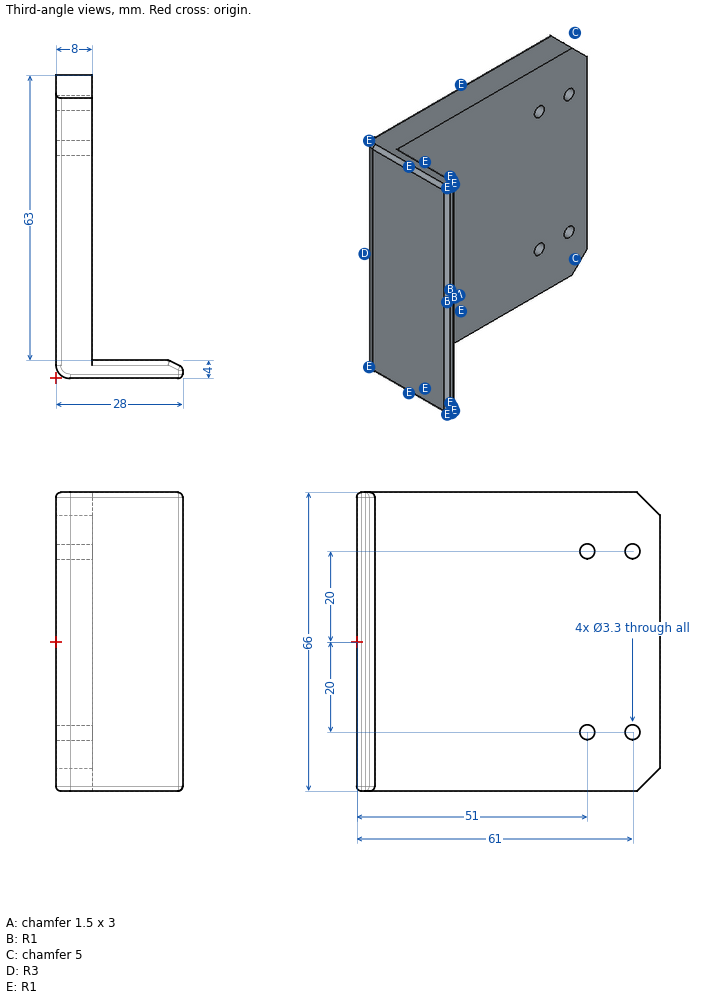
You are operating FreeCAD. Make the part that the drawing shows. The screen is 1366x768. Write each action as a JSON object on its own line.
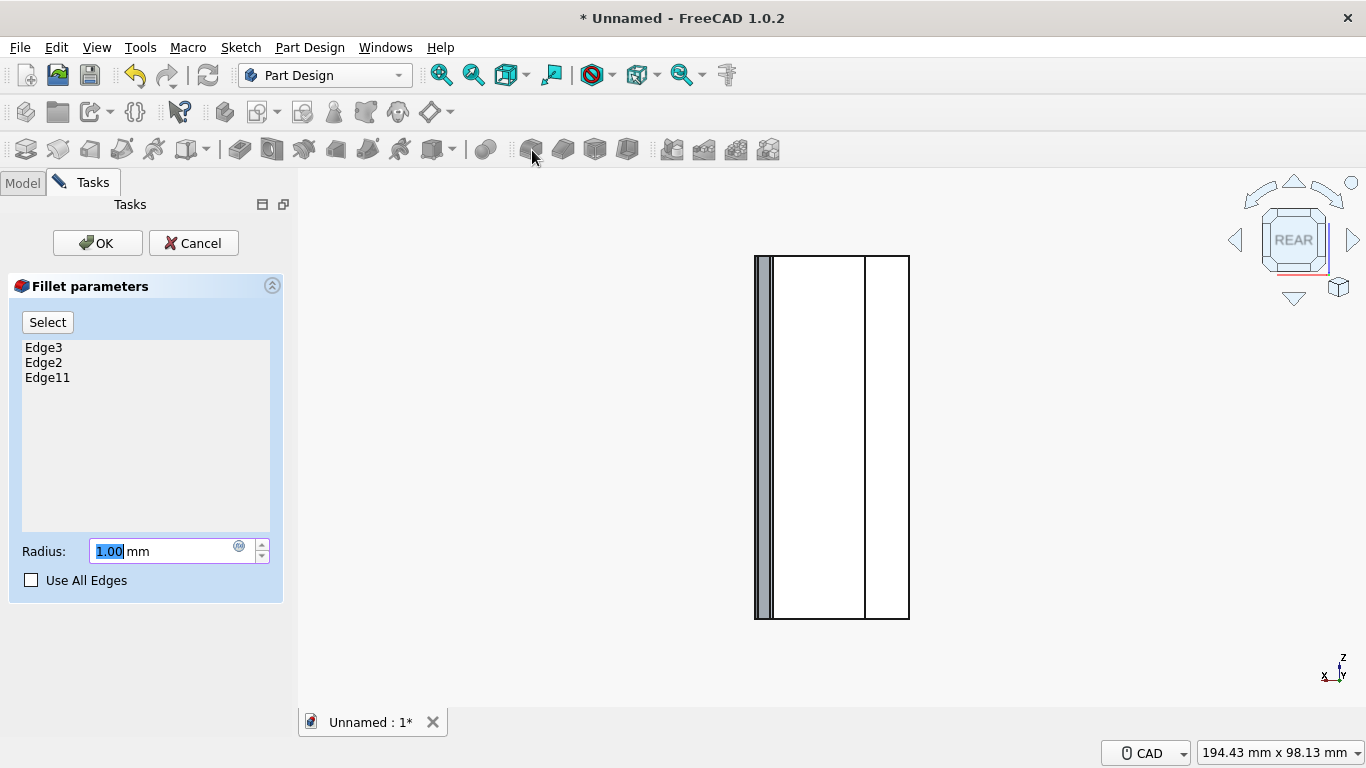
{"action": "type", "text": "1"}
{"action": "key", "text": "Tab"}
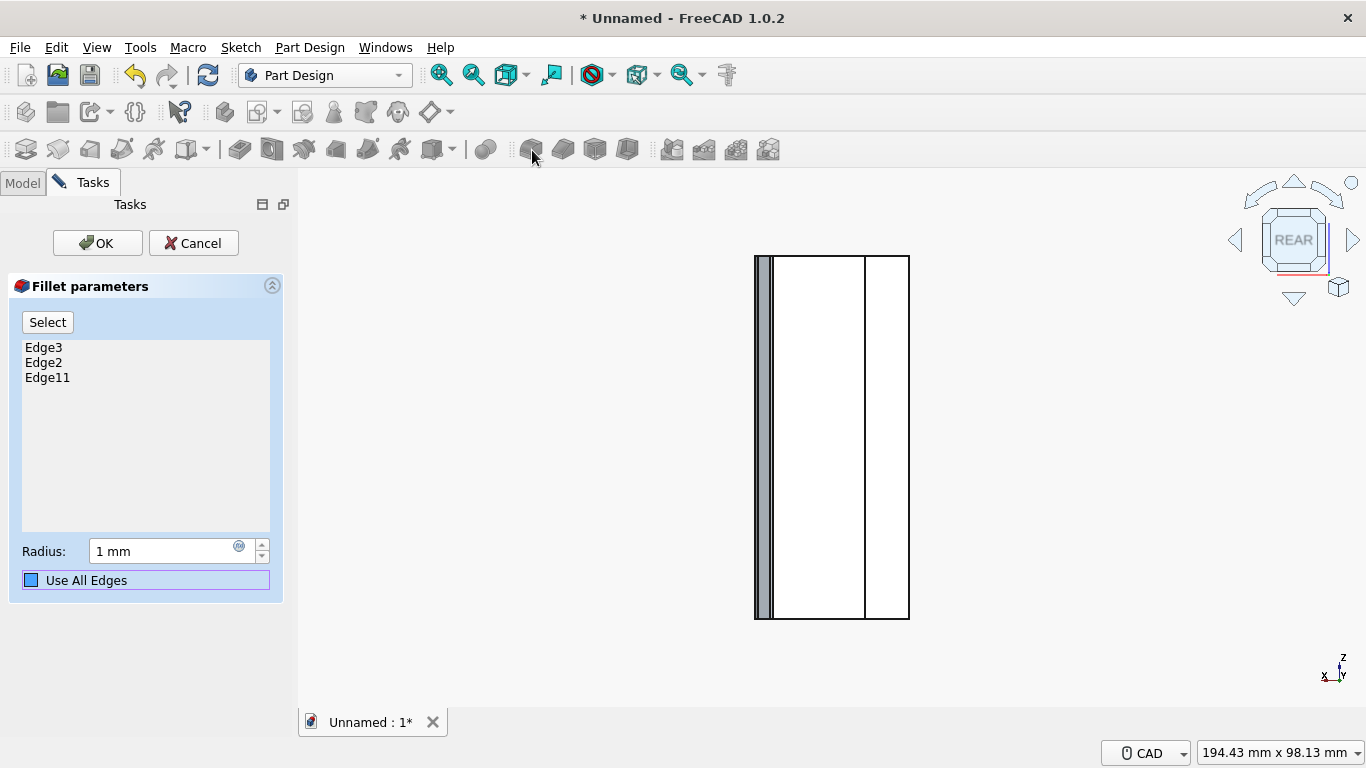
{"action": "left_click", "coordinate": [98, 243]}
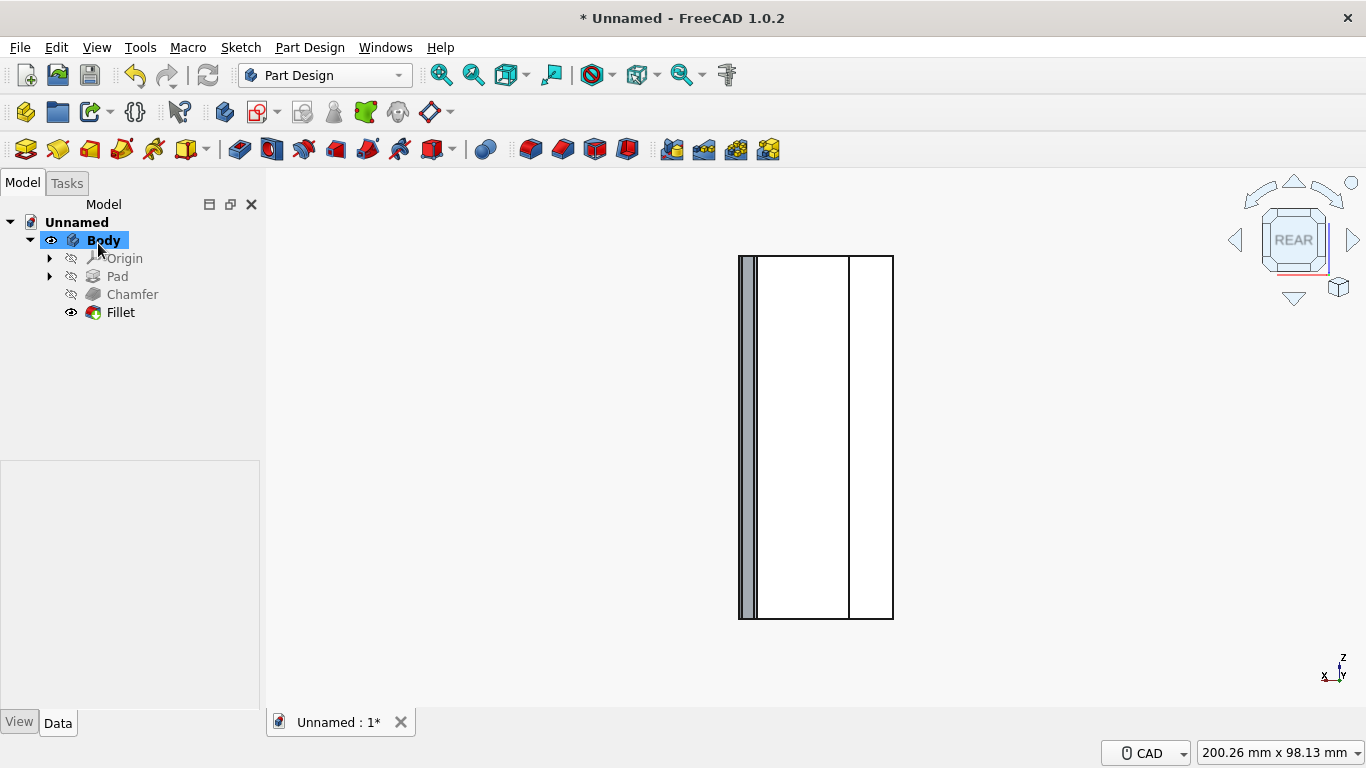
{"action": "left_click", "coordinate": [871, 255]}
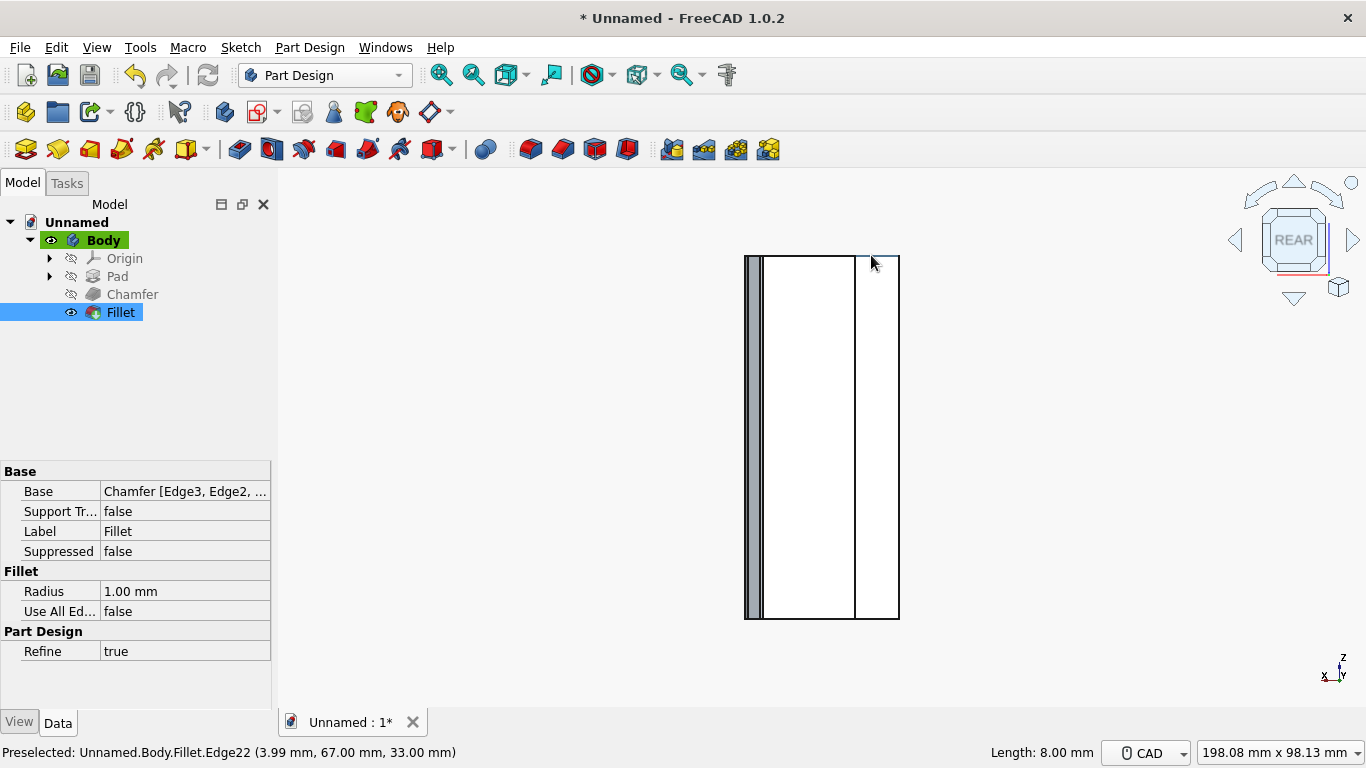
{"action": "left_click", "coordinate": [877, 618], "text": "ctrl"}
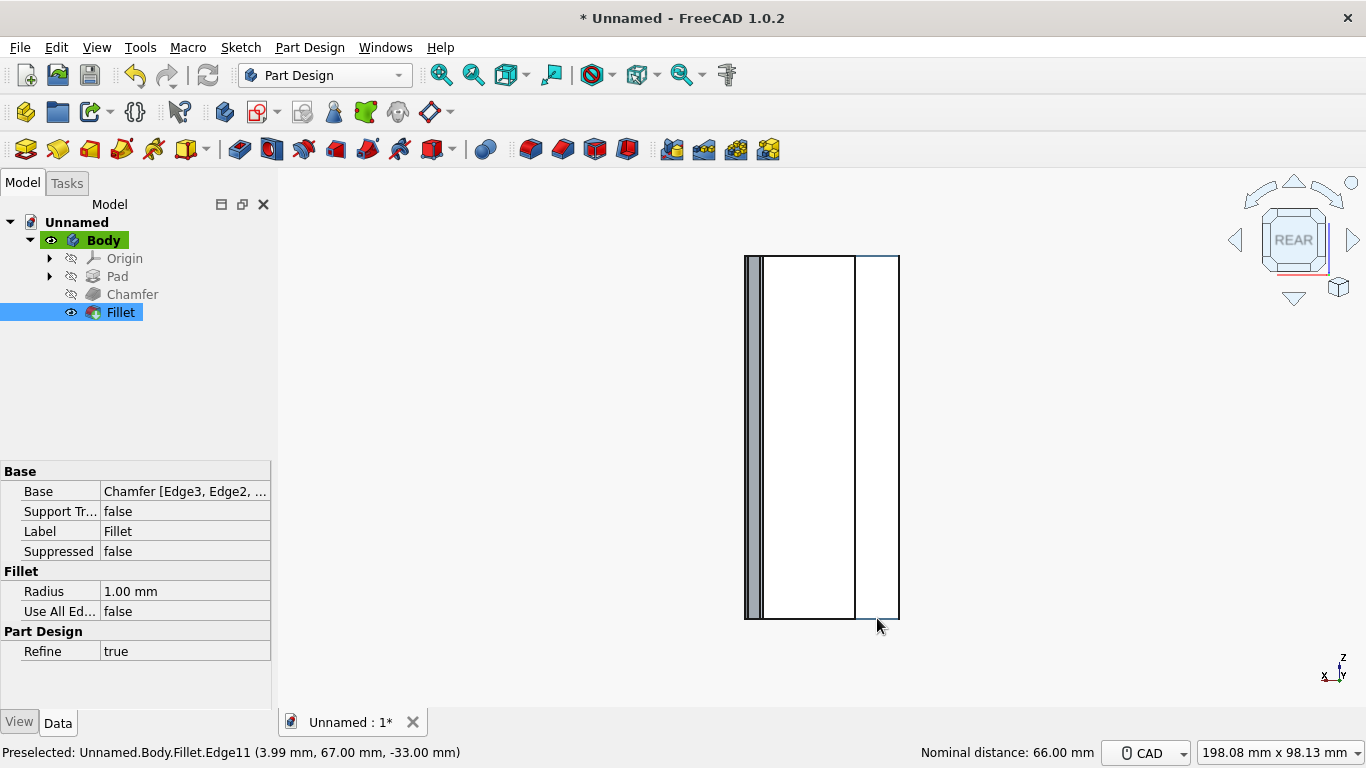
{"action": "left_click", "coordinate": [564, 150]}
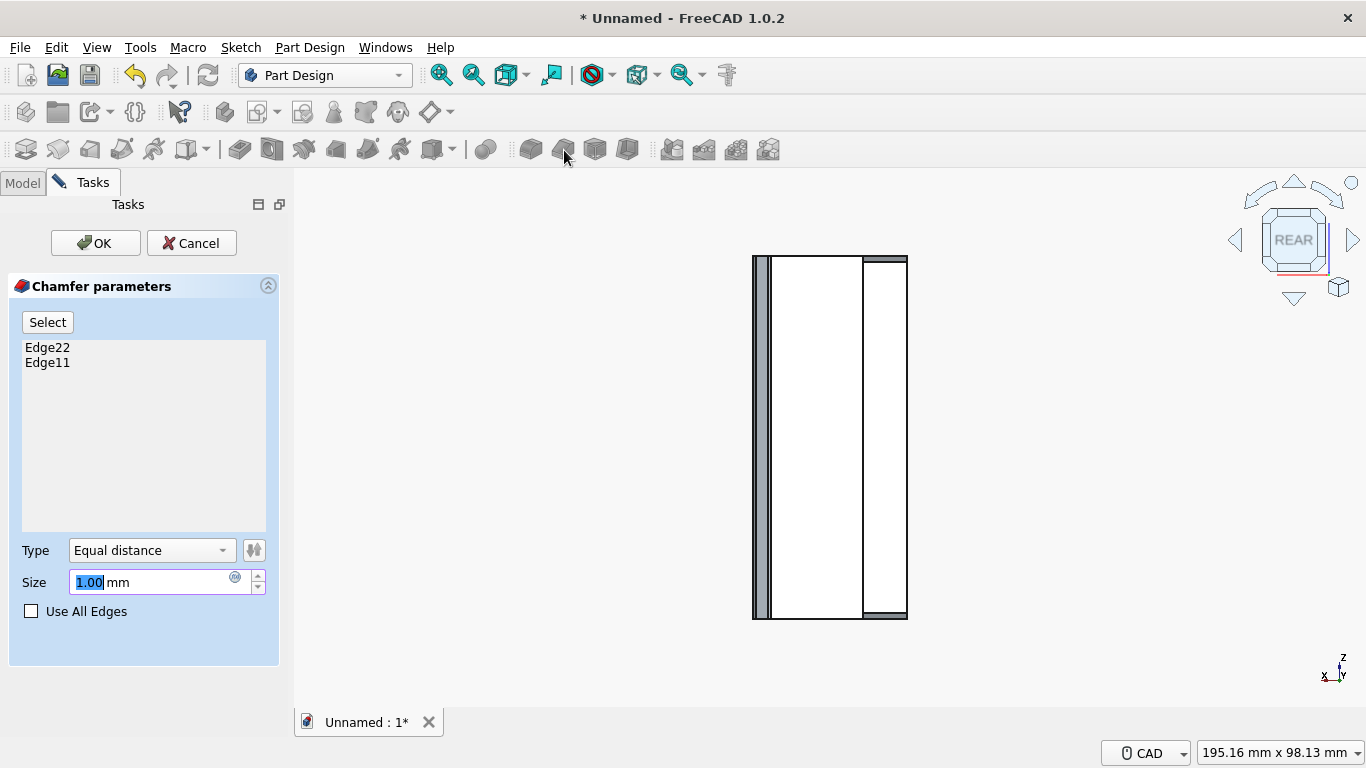
{"action": "type", "text": "5"}
{"action": "key", "text": "Tab"}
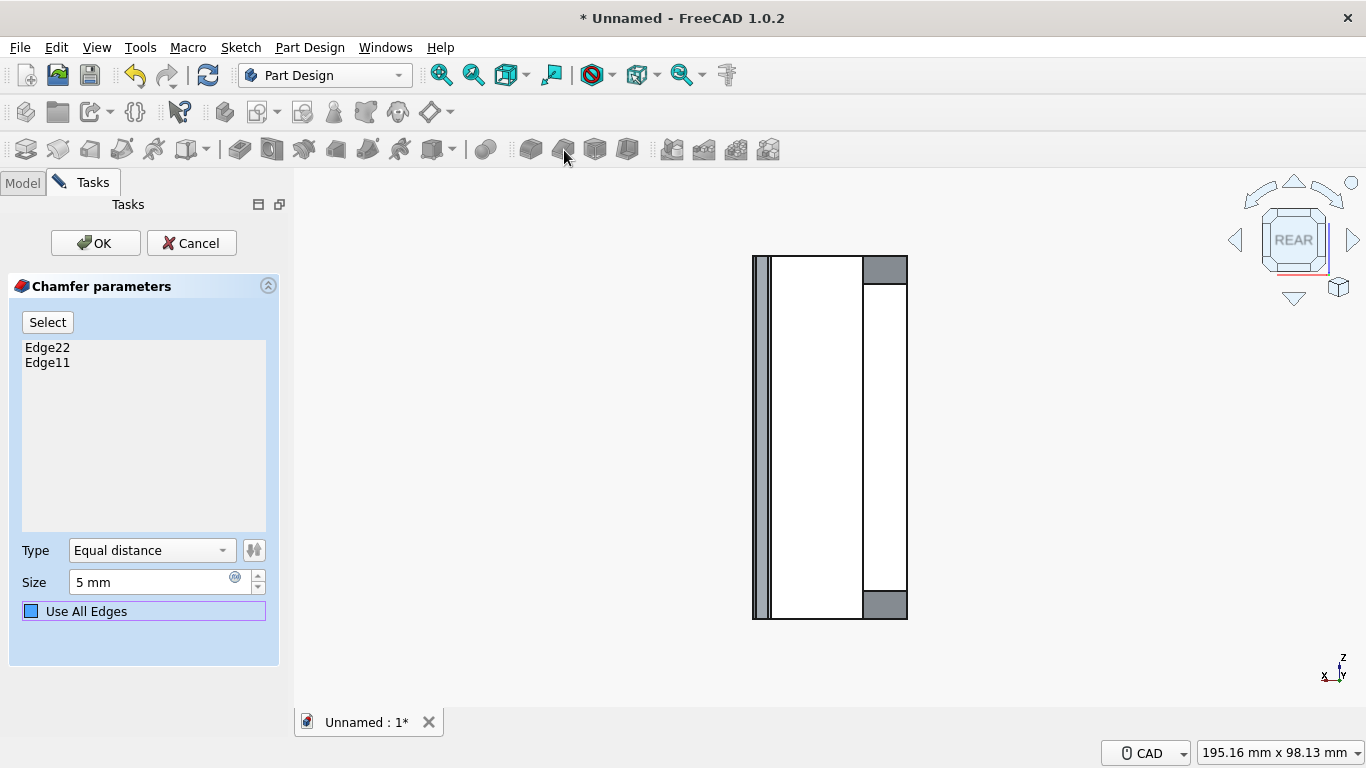
{"action": "left_click", "coordinate": [96, 243]}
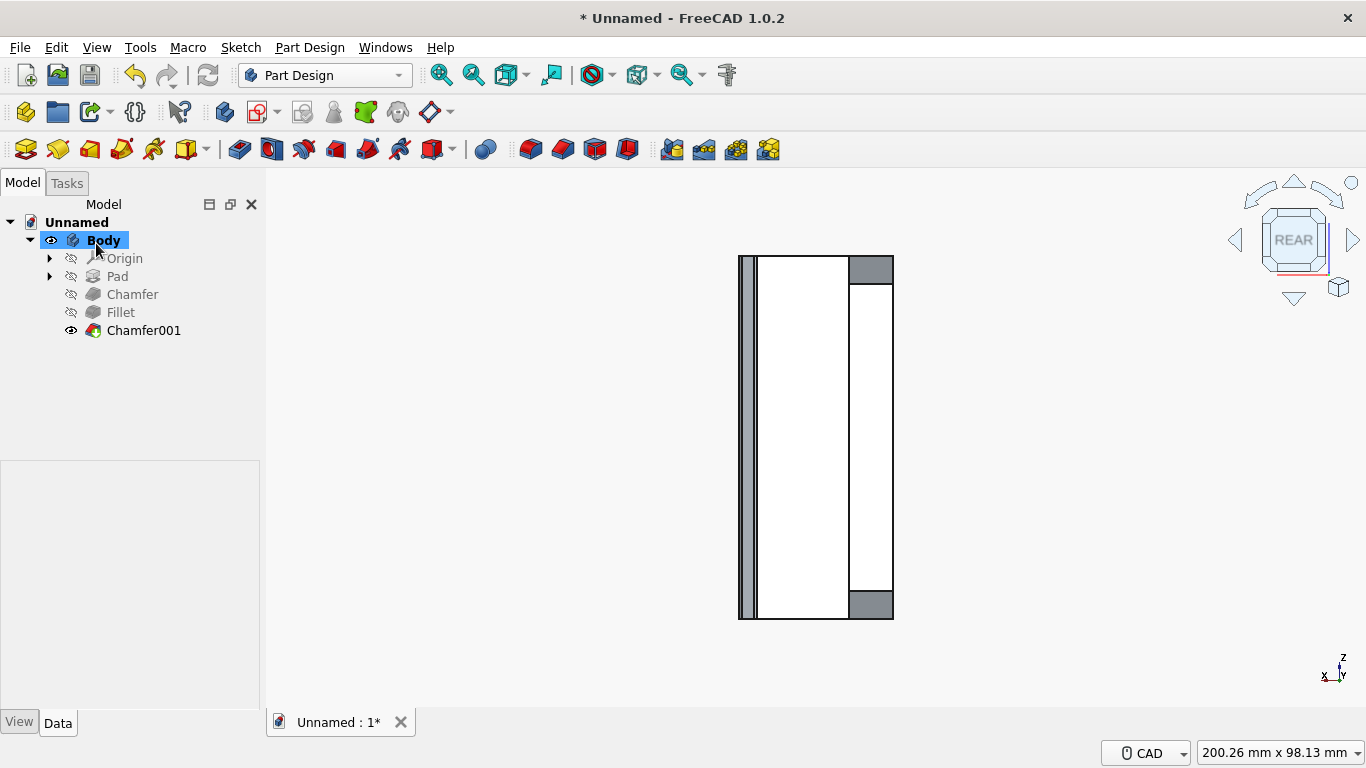
{"action": "key", "text": "0"}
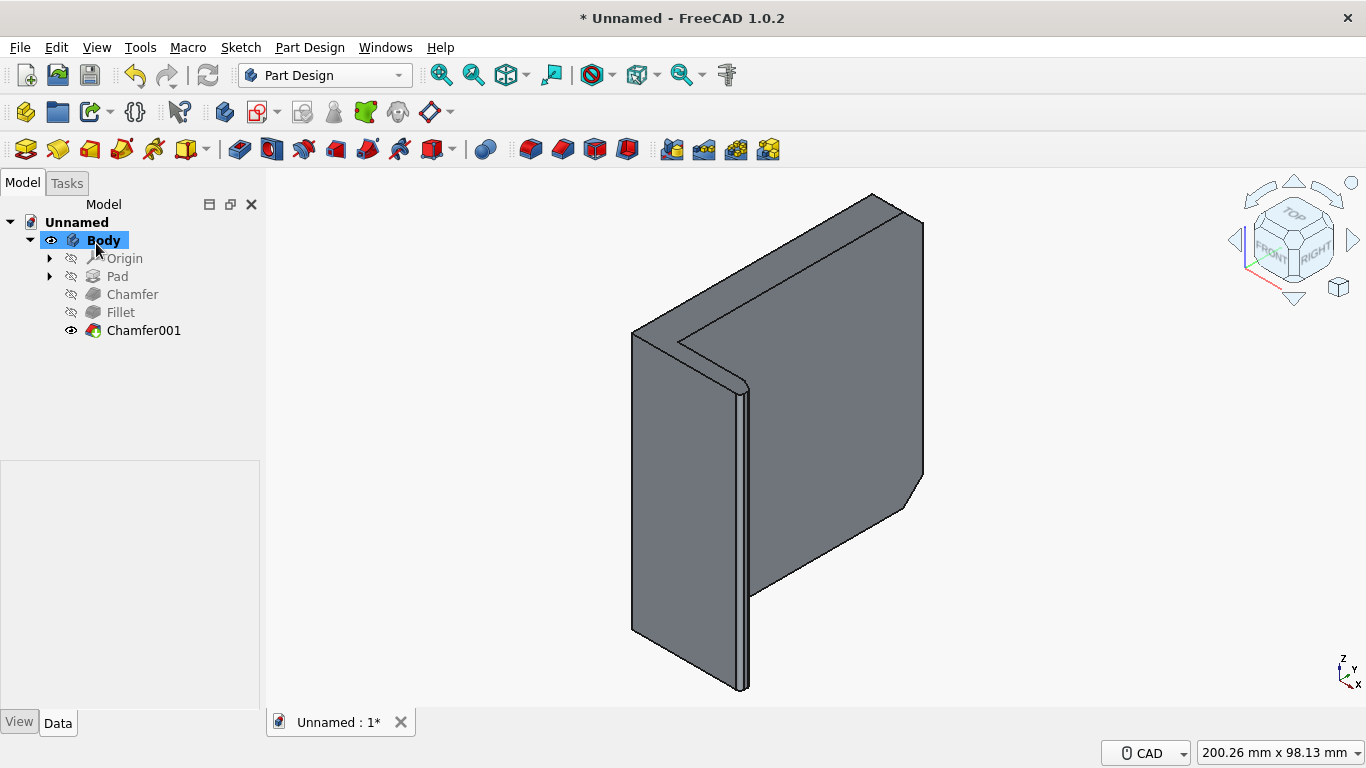
{"action": "key", "text": "2"}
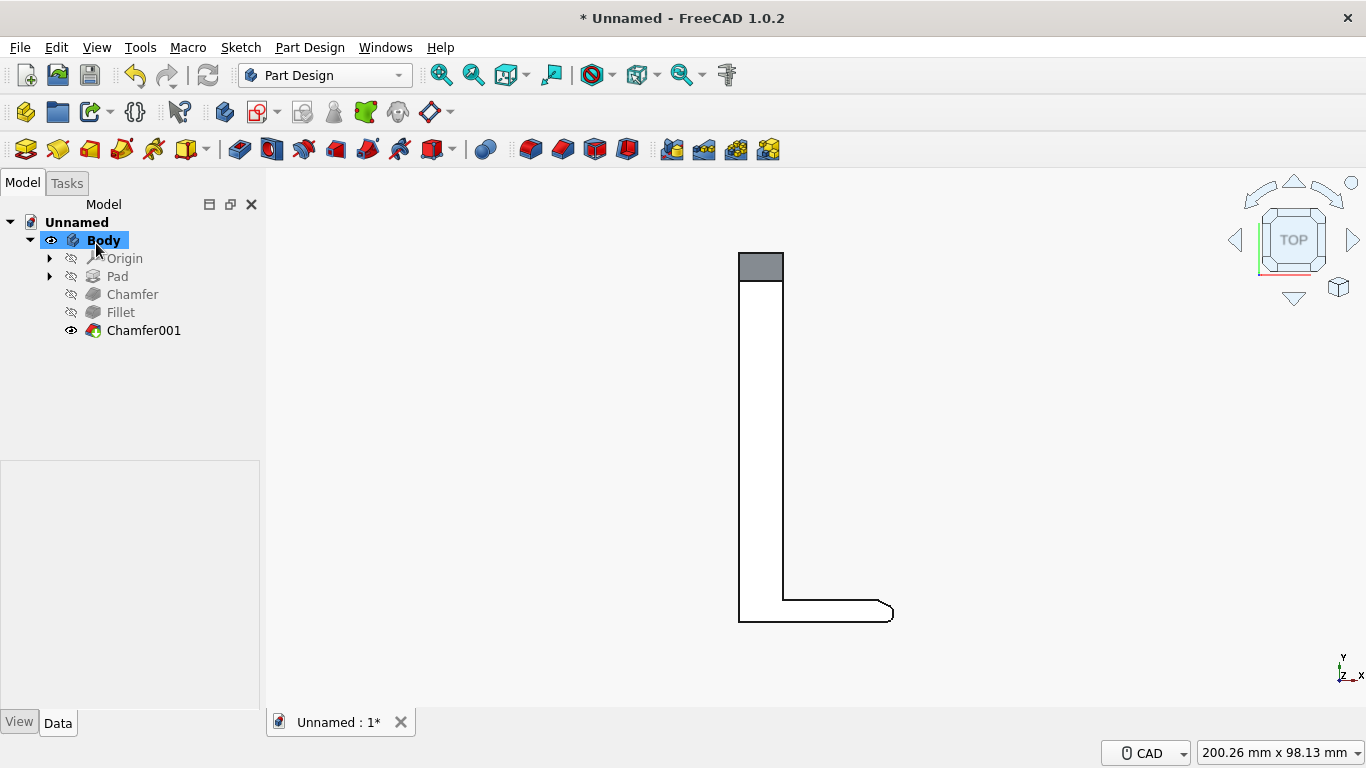
{"action": "key", "text": "1"}